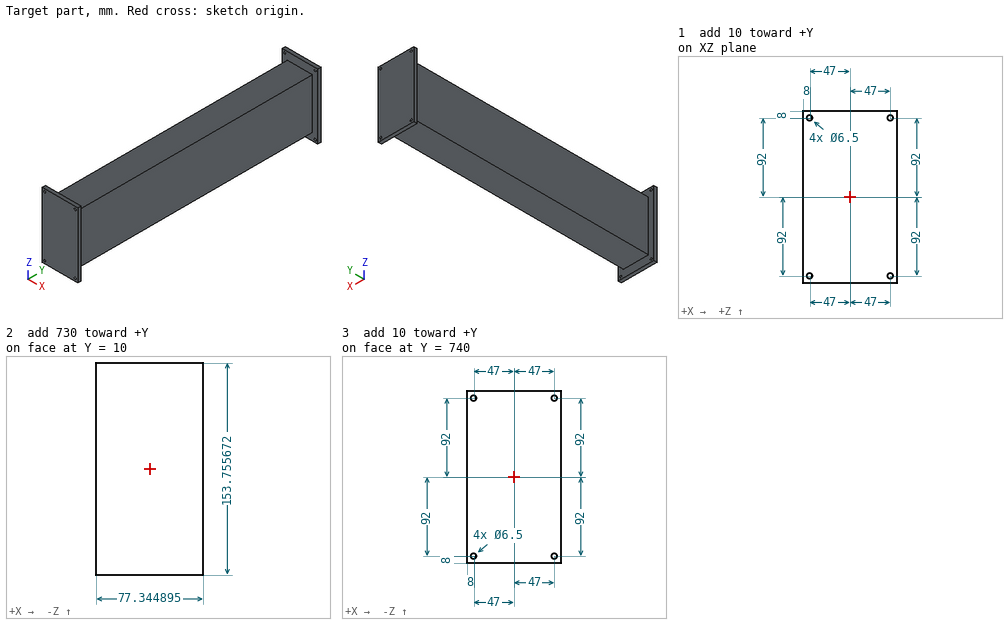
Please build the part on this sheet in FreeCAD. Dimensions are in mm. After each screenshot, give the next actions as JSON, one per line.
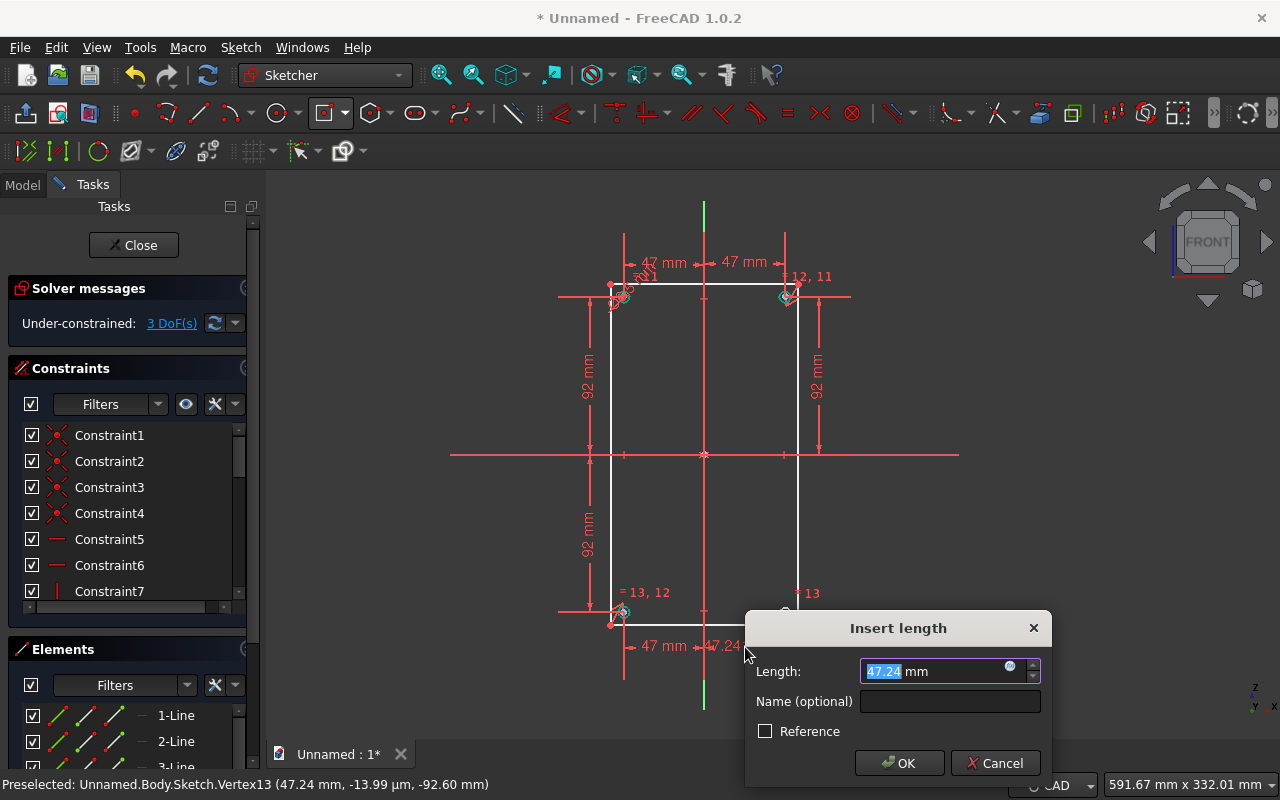
{"action": "type", "text": "47"}
{"action": "key", "text": "Return"}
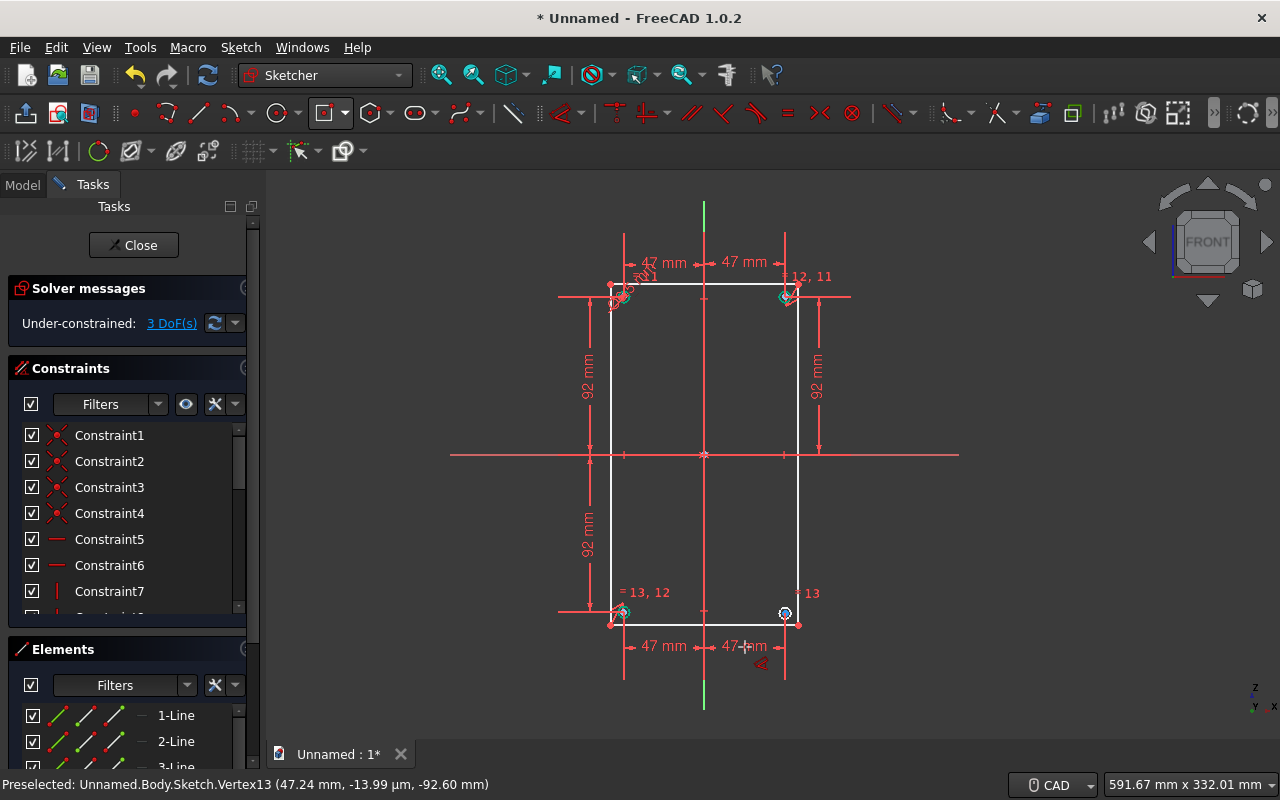
{"action": "left_click", "coordinate": [785, 613]}
{"action": "left_click", "coordinate": [819, 534]}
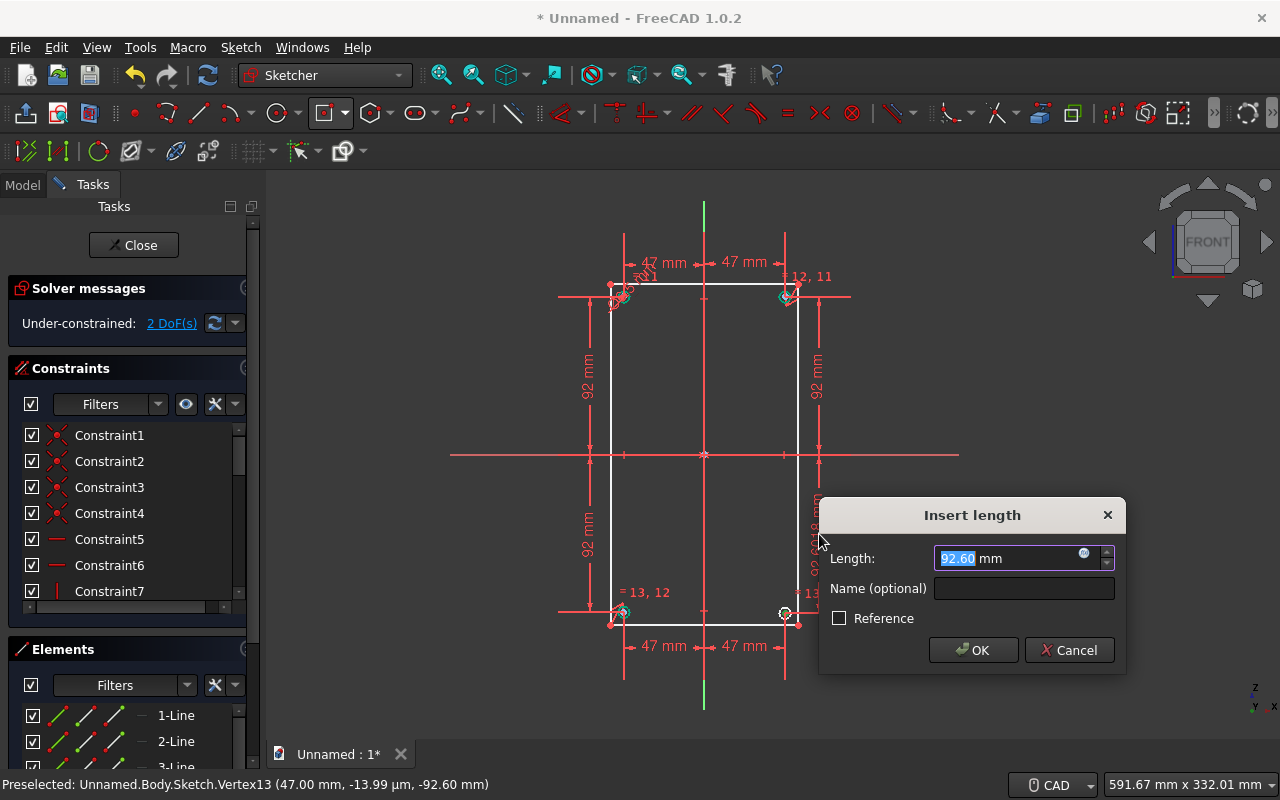
{"action": "type", "text": "92"}
{"action": "key", "text": "Return"}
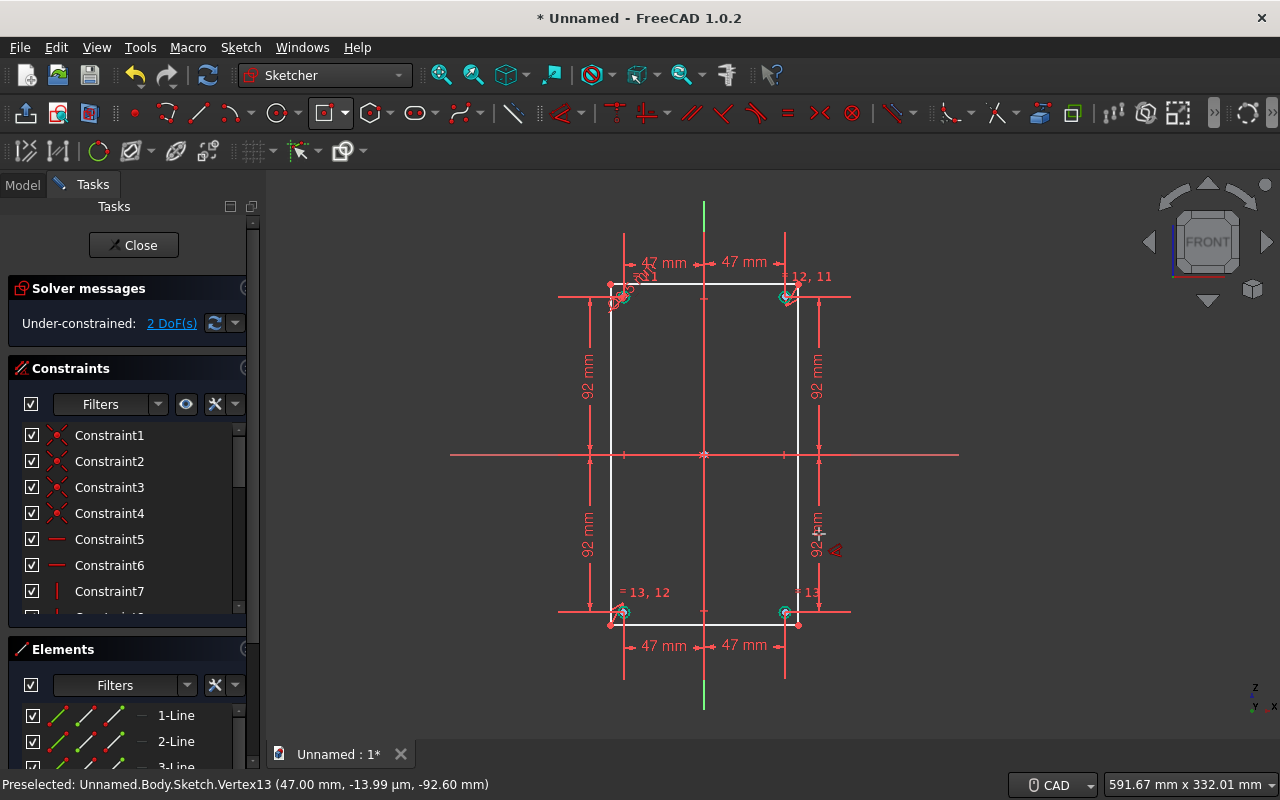
{"action": "scroll", "coordinate": [611, 284], "scroll_direction": "up", "scroll_amount": 6}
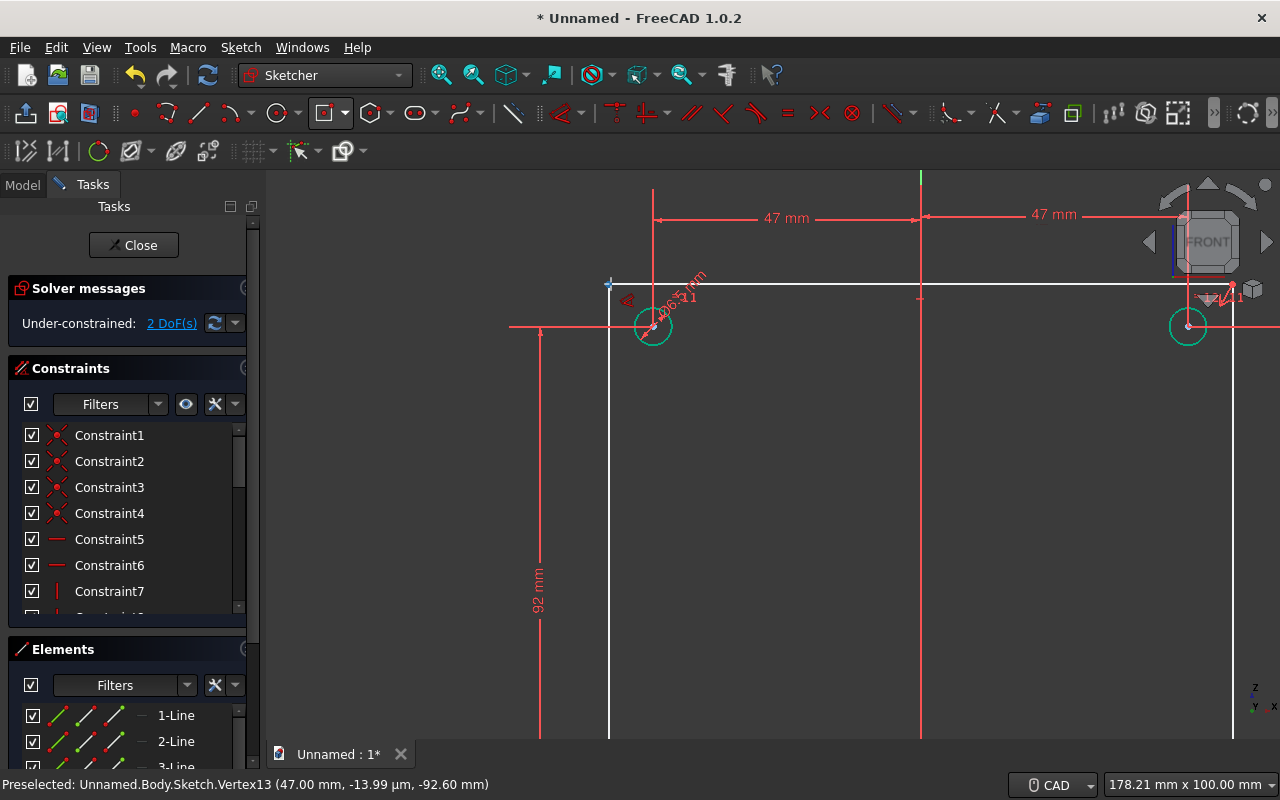
{"action": "left_click", "coordinate": [609, 284]}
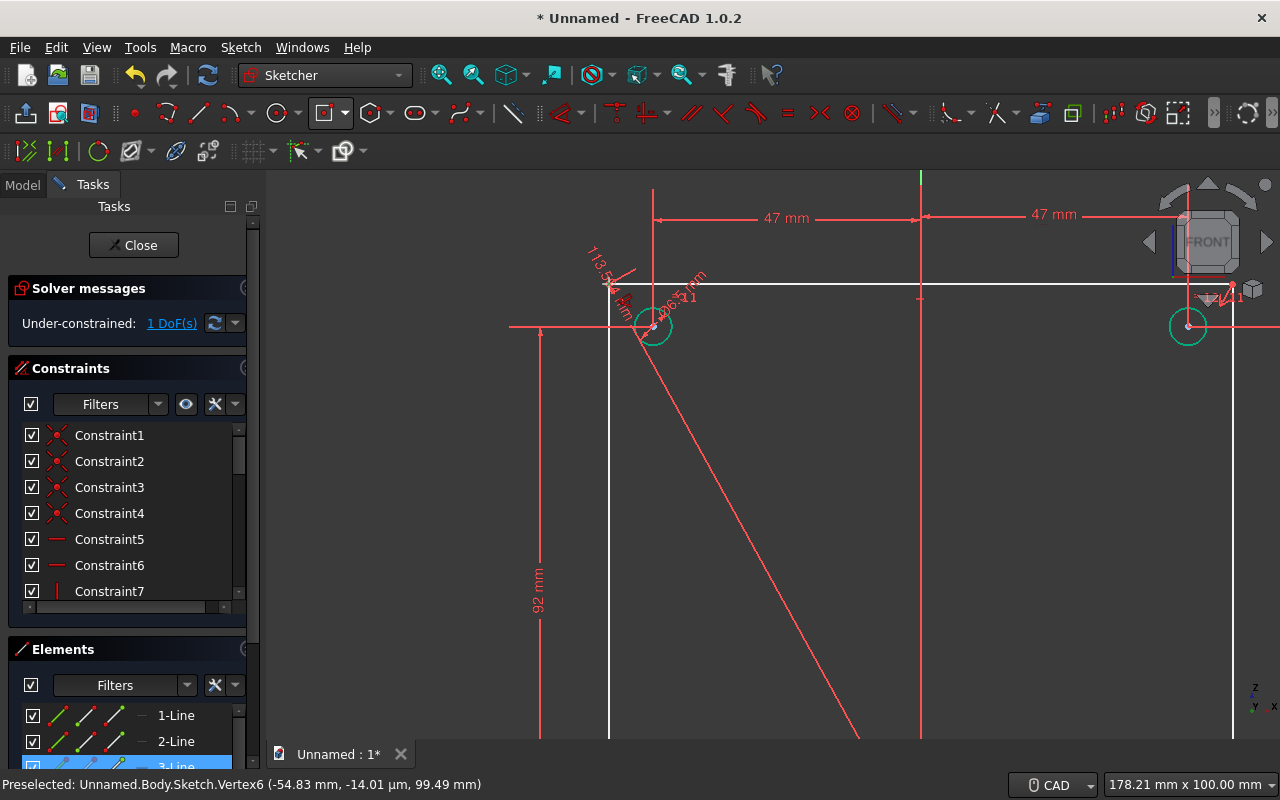
{"action": "left_click", "coordinate": [653, 327]}
{"action": "left_click", "coordinate": [631, 250]}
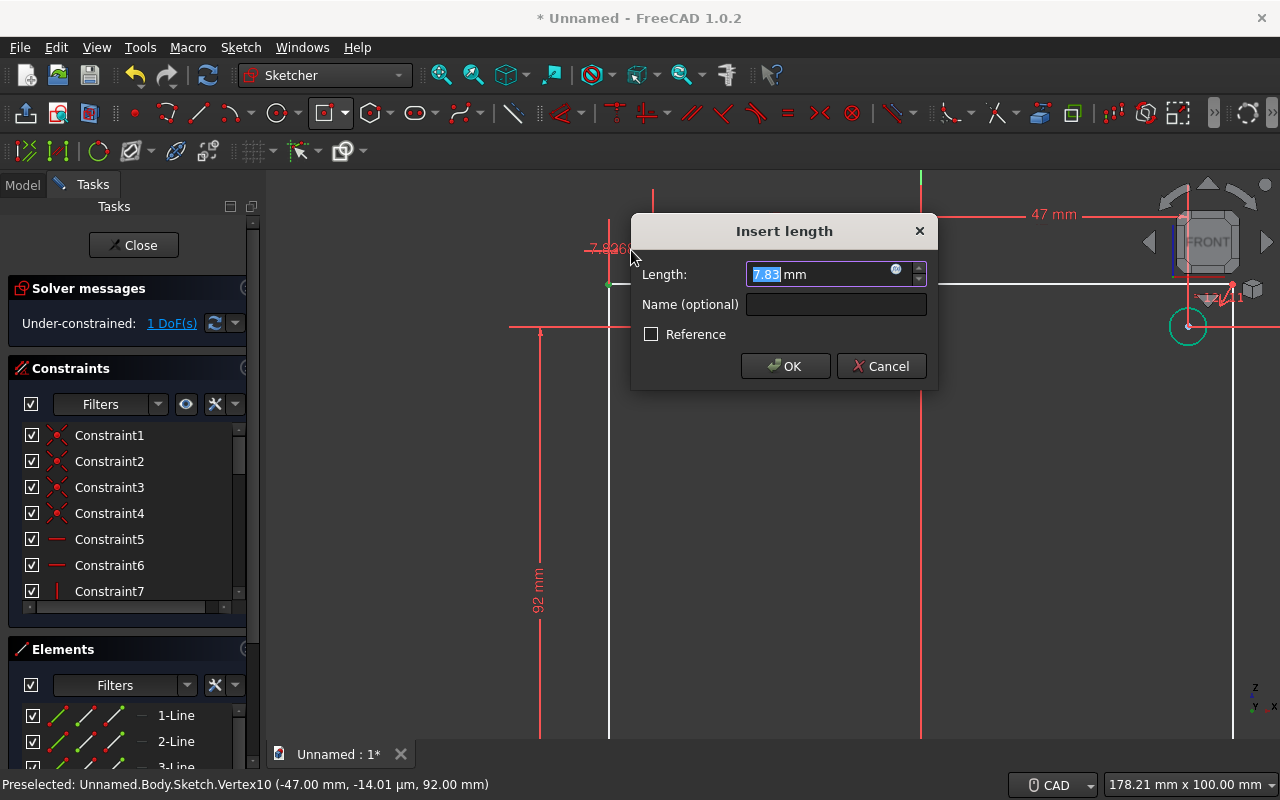
{"action": "type", "text": "8"}
{"action": "key", "text": "Return"}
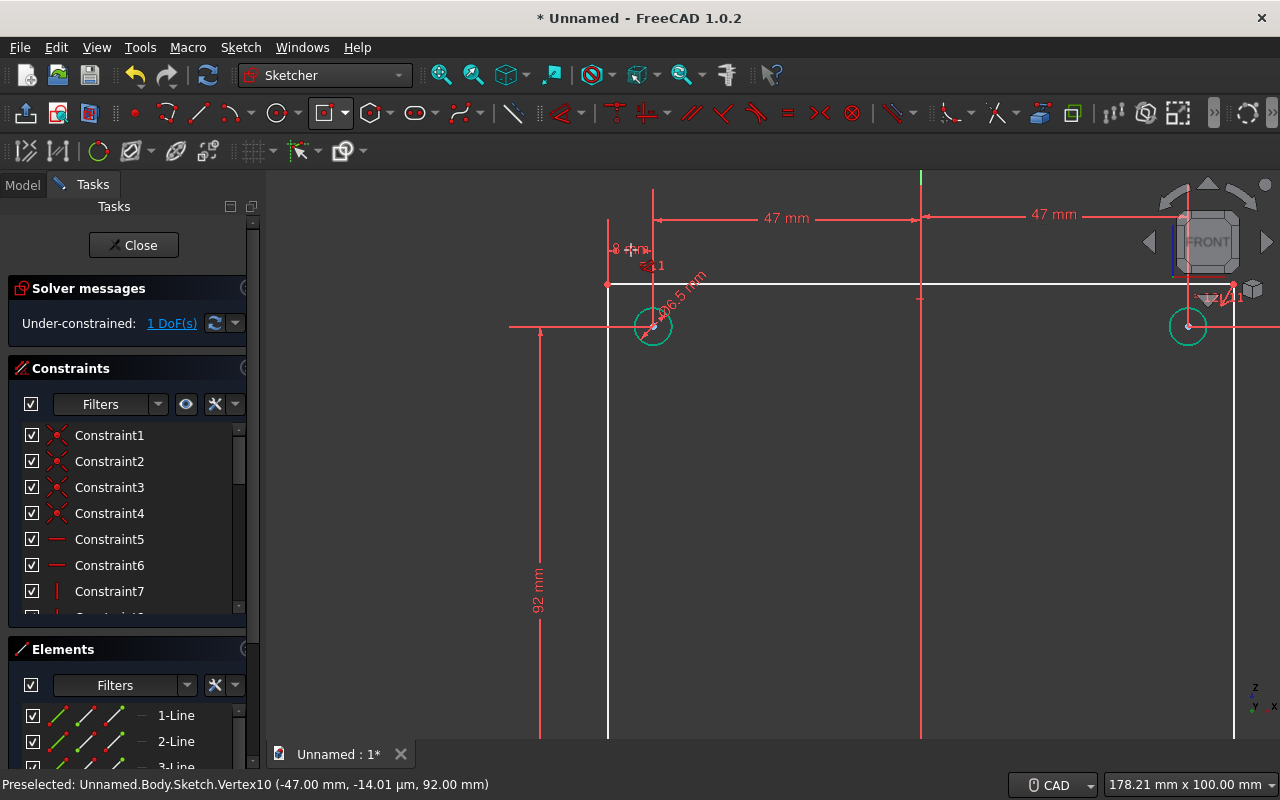
{"action": "left_click", "coordinate": [608, 284]}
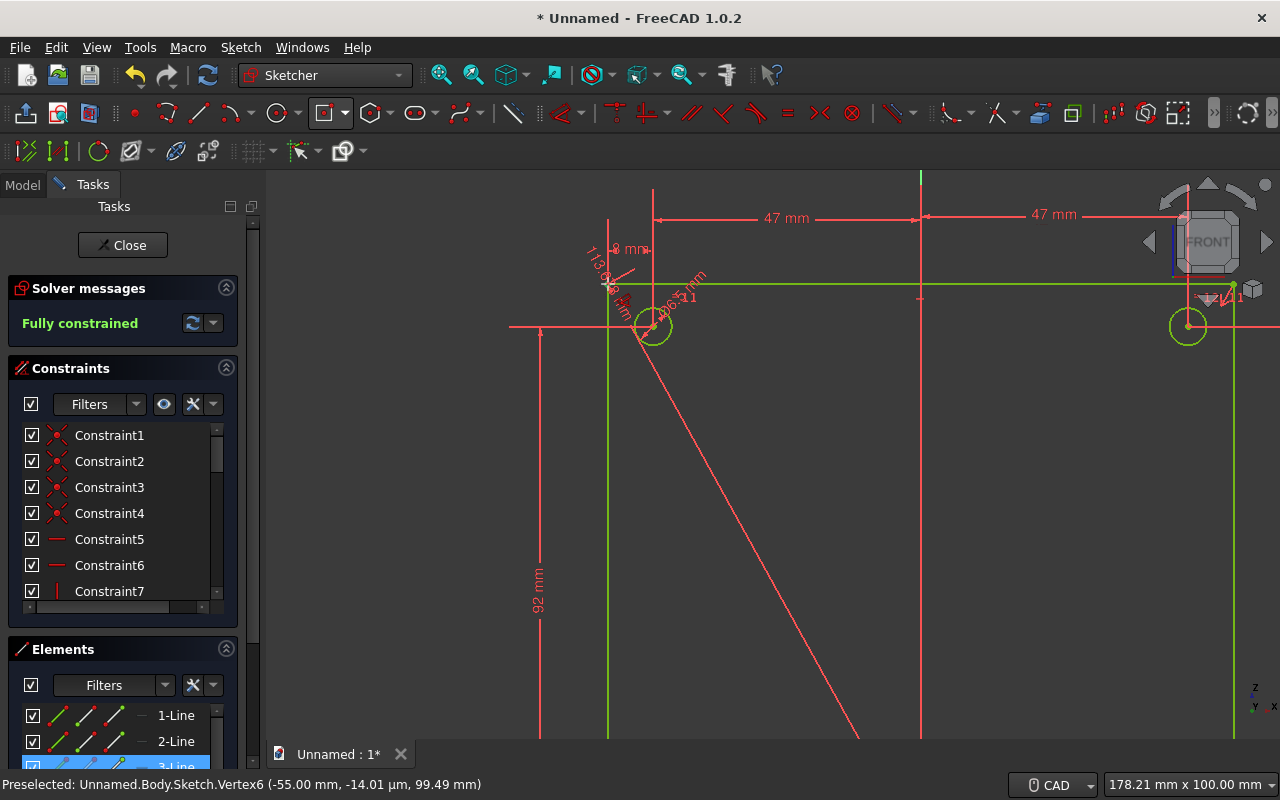
{"action": "left_click", "coordinate": [653, 327]}
{"action": "left_click", "coordinate": [574, 305]}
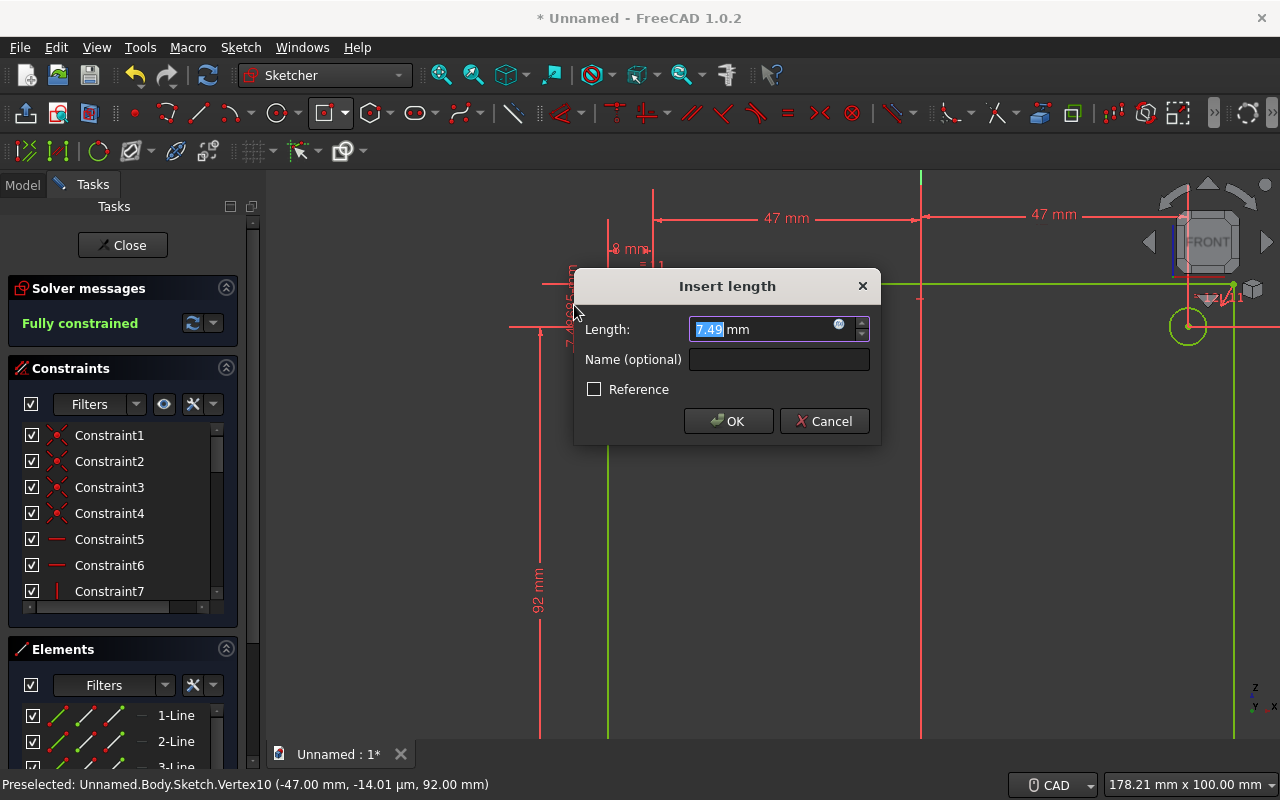
{"action": "type", "text": "8"}
{"action": "key", "text": "Return"}
{"action": "key", "text": "Escape"}